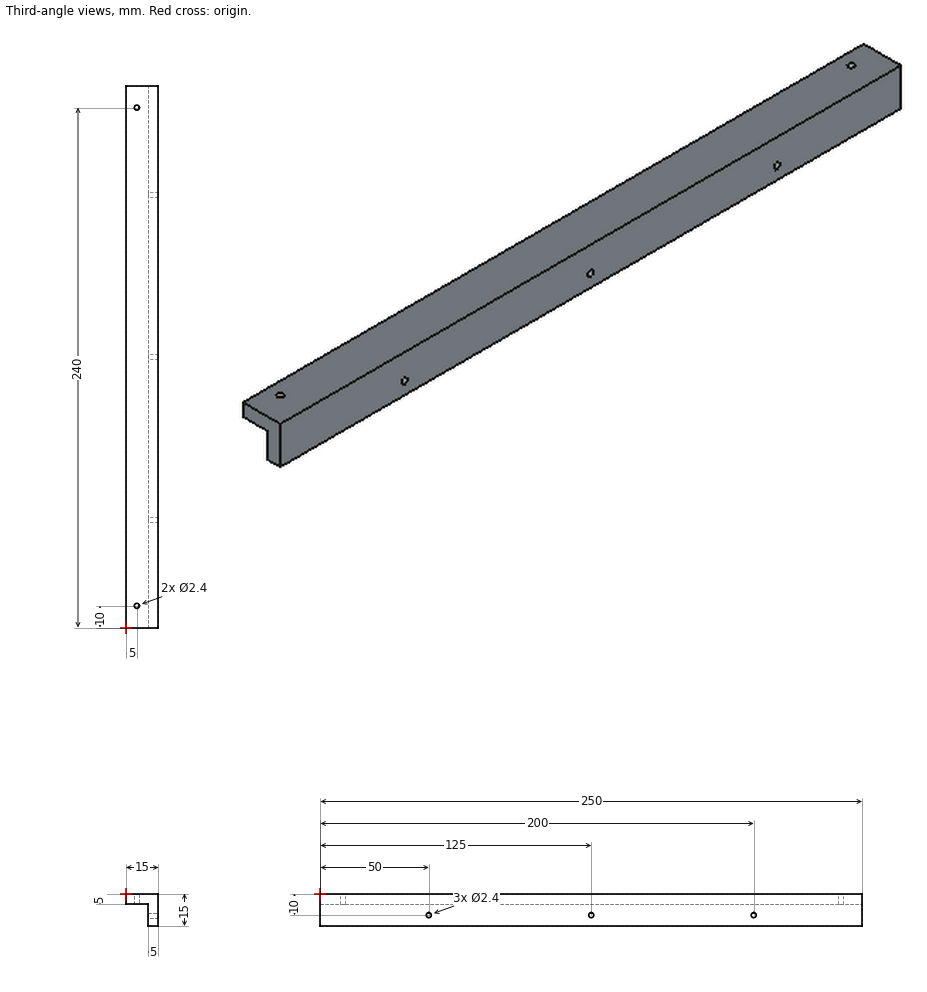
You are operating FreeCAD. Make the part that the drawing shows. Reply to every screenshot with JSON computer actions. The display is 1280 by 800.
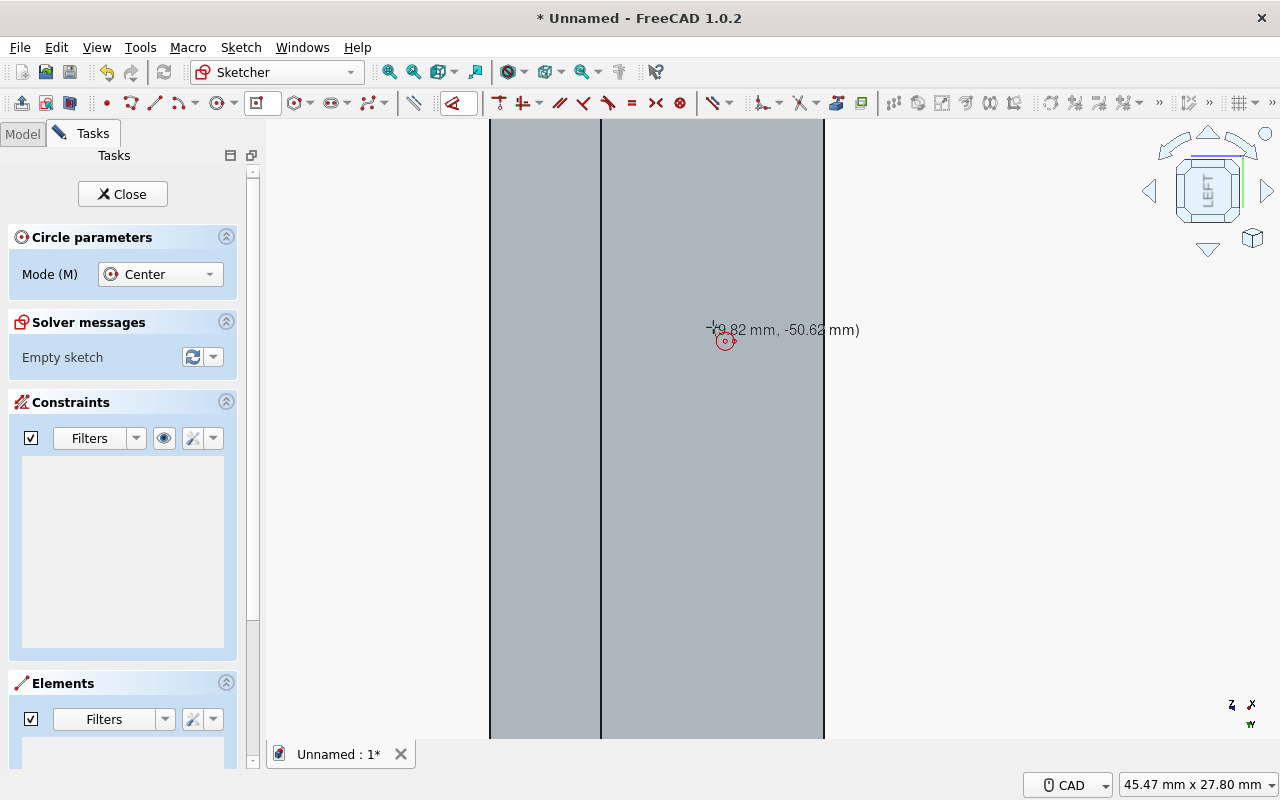
{"action": "scroll", "coordinate": [713, 327], "scroll_direction": "down", "scroll_amount": 12}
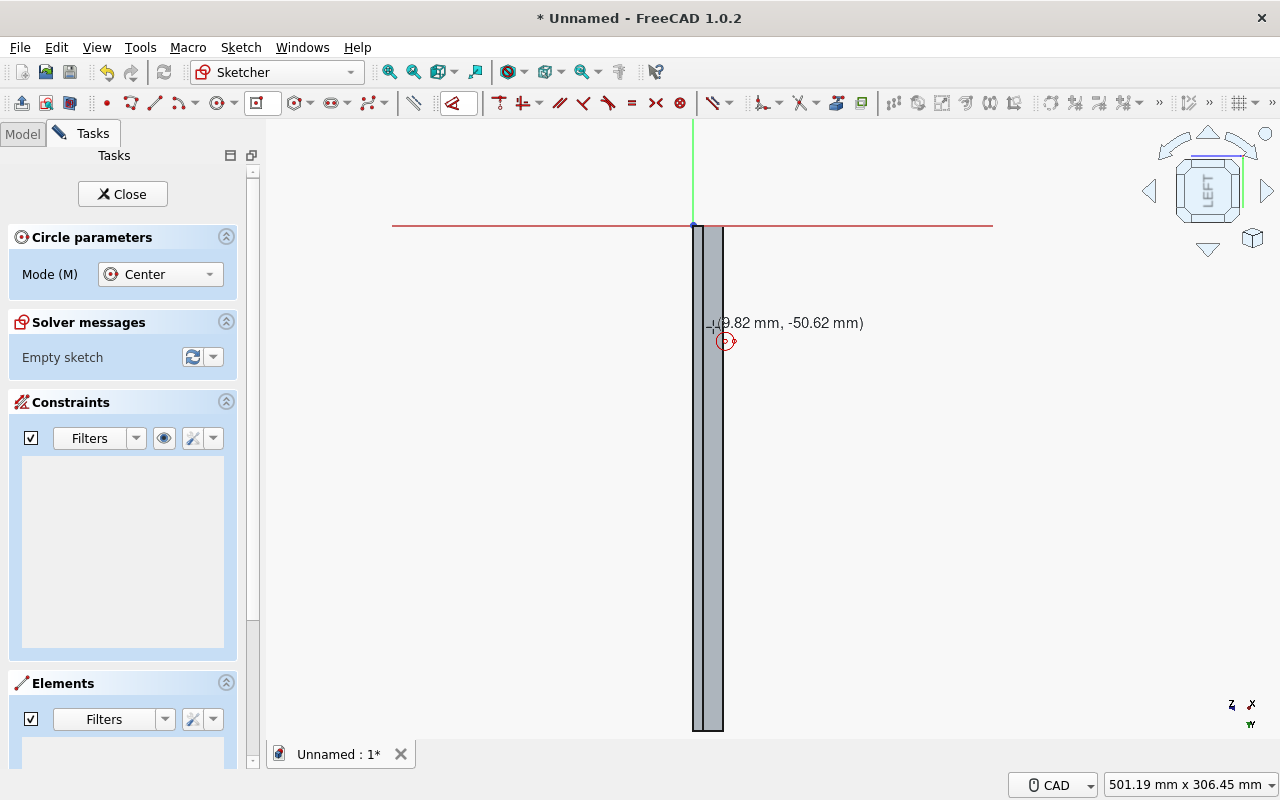
{"action": "left_click", "coordinate": [713, 327]}
{"action": "mouse_move", "coordinate": [715, 325]}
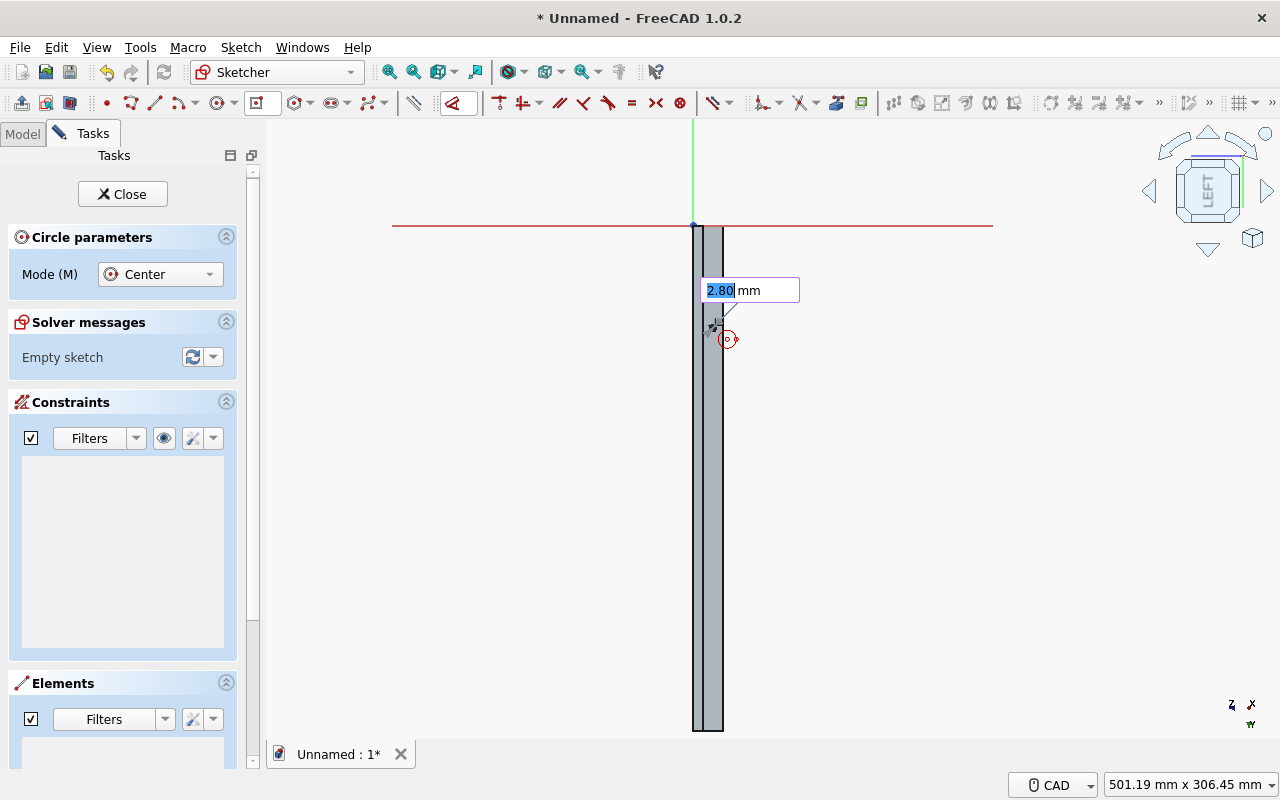
{"action": "type", "text": "2.4"}
{"action": "key", "text": "Return"}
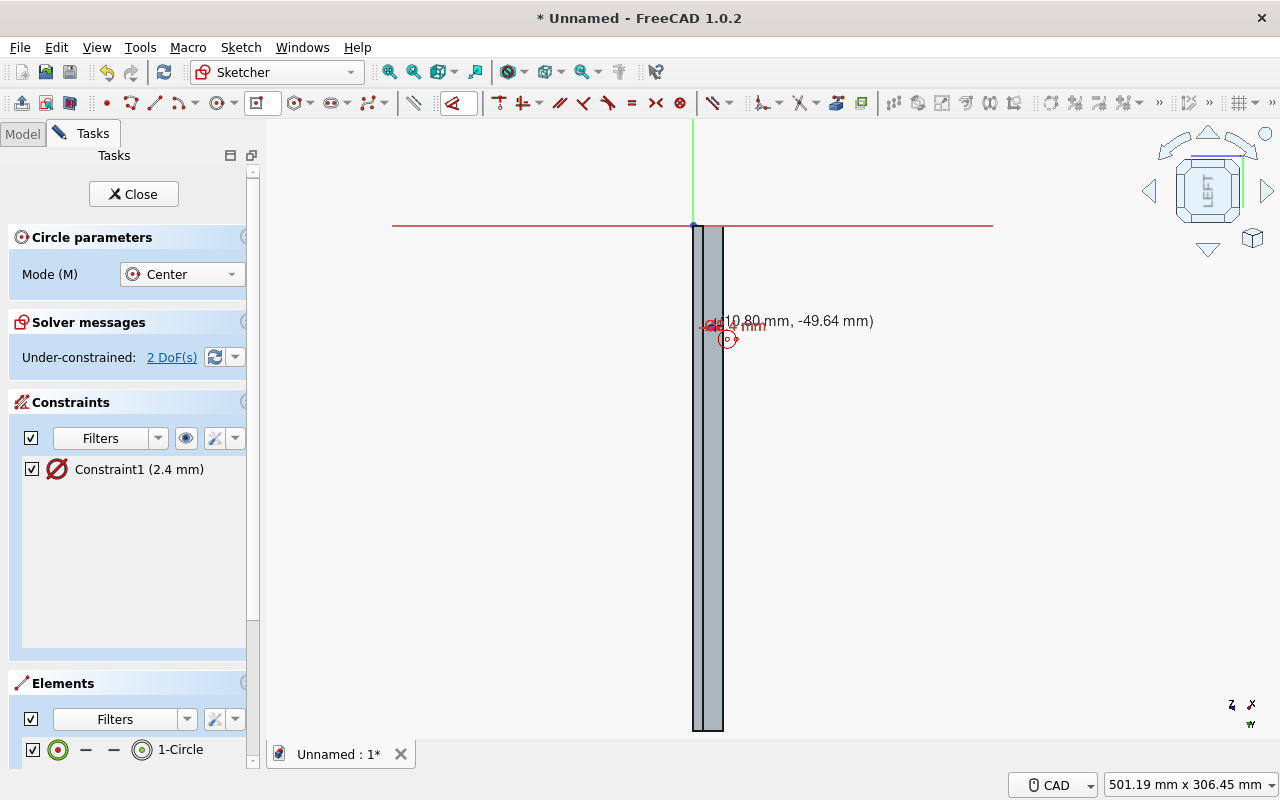
{"action": "scroll", "coordinate": [713, 478], "scroll_direction": "up", "scroll_amount": 12}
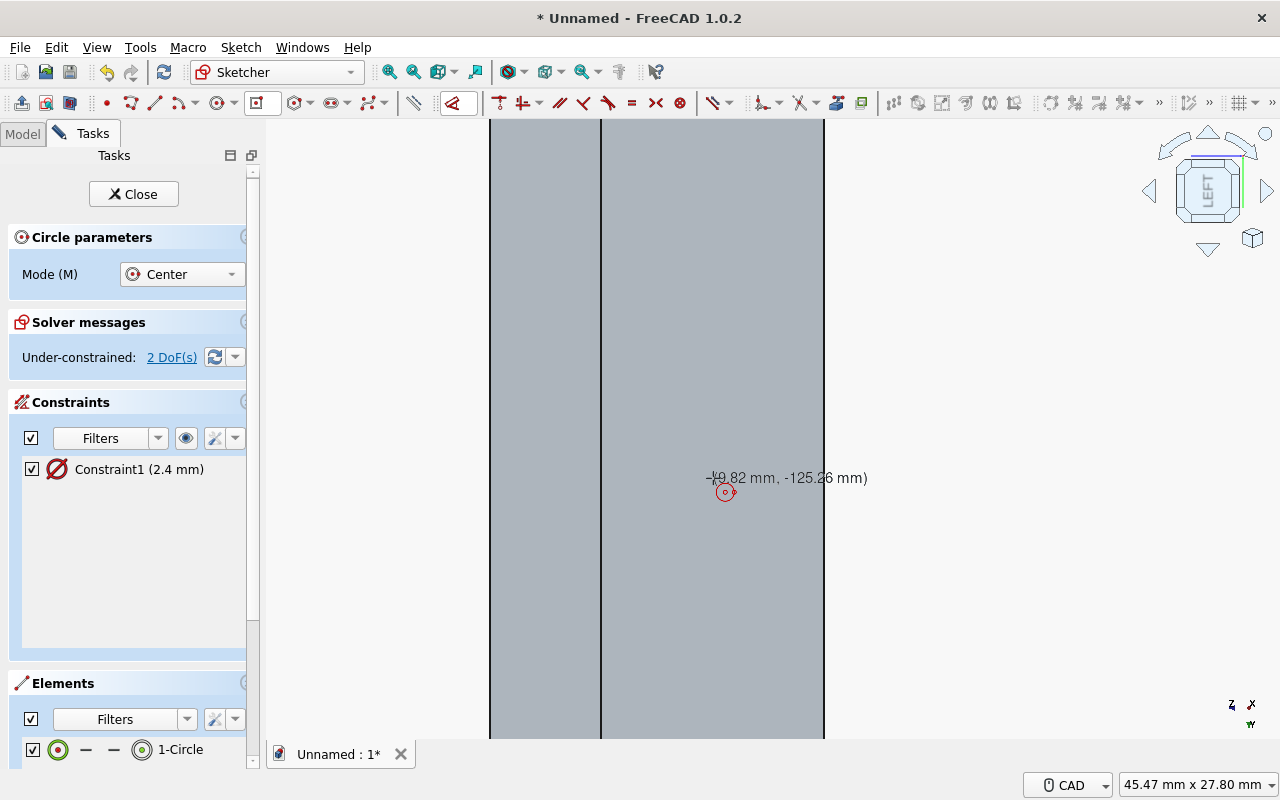
{"action": "scroll", "coordinate": [713, 478], "scroll_direction": "down", "scroll_amount": 12}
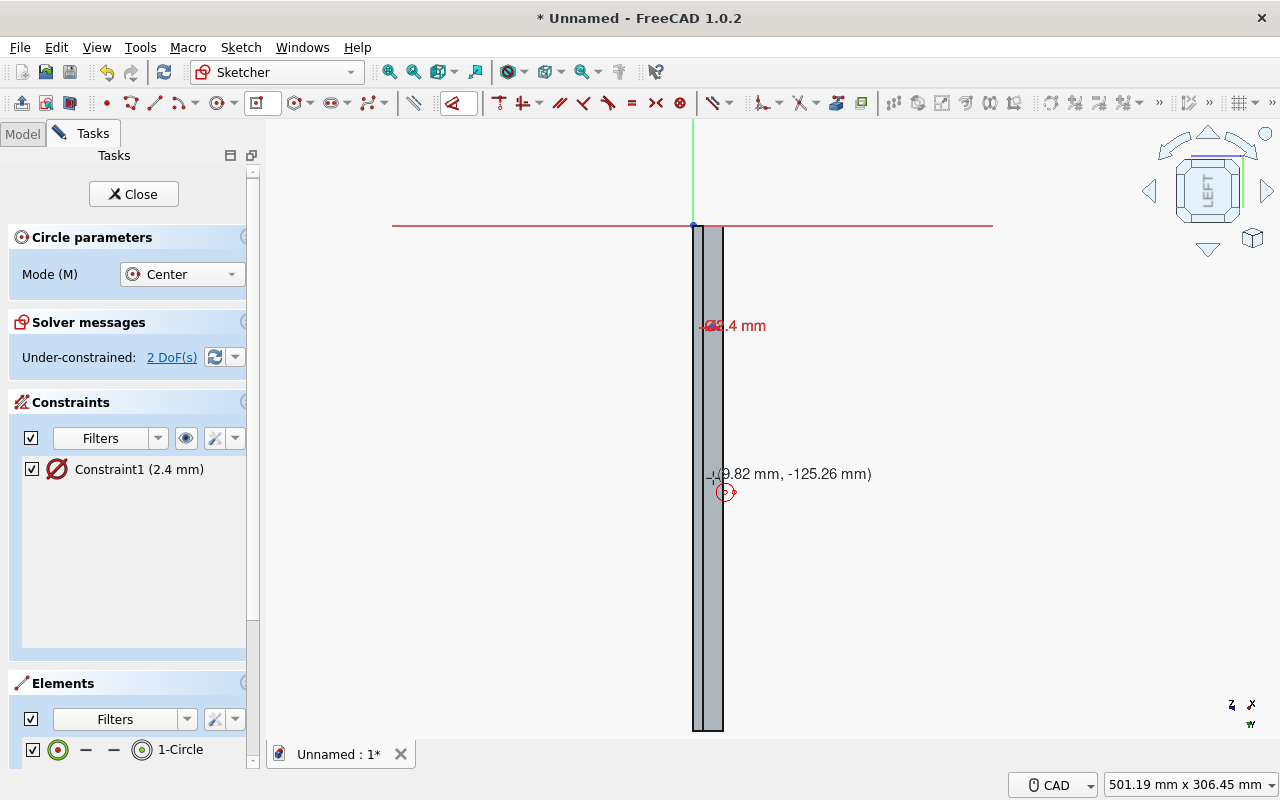
{"action": "left_click", "coordinate": [713, 478]}
{"action": "mouse_move", "coordinate": [715, 477]}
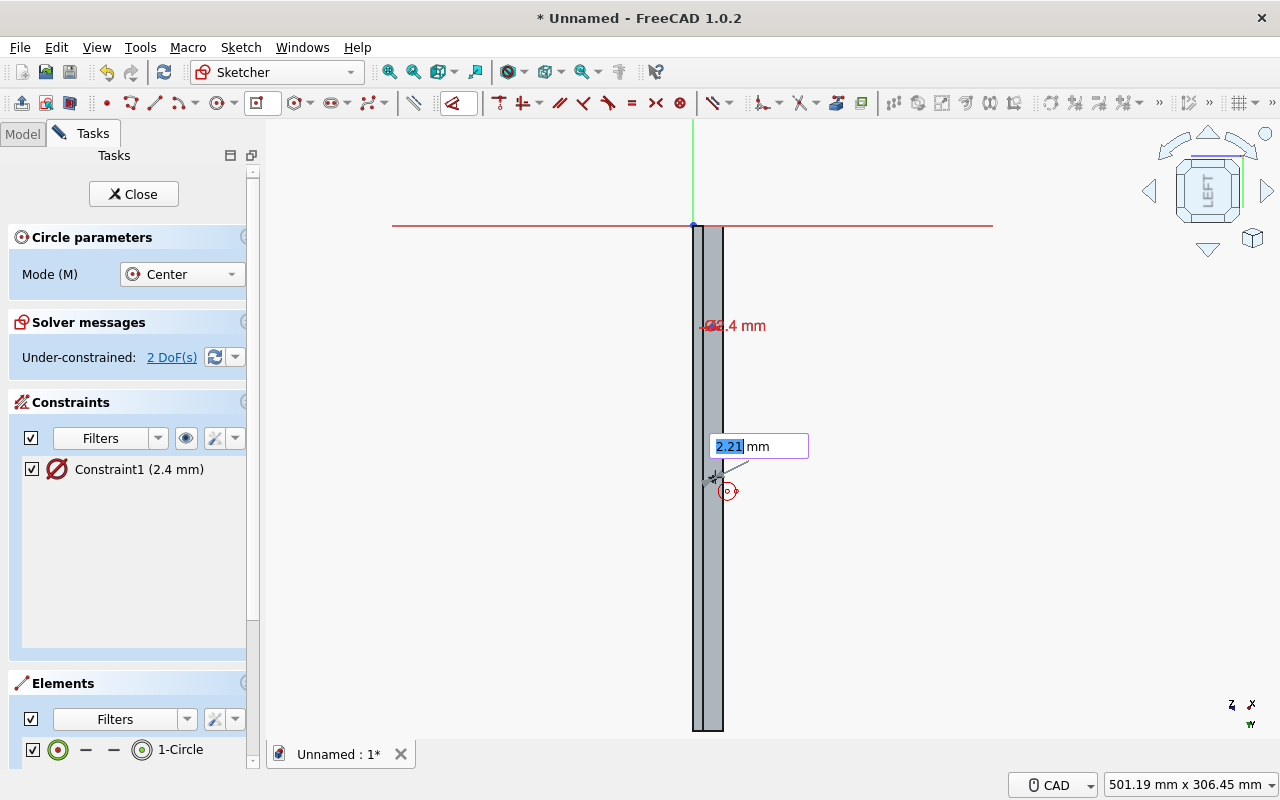
{"action": "type", "text": "2.4"}
{"action": "key", "text": "Return"}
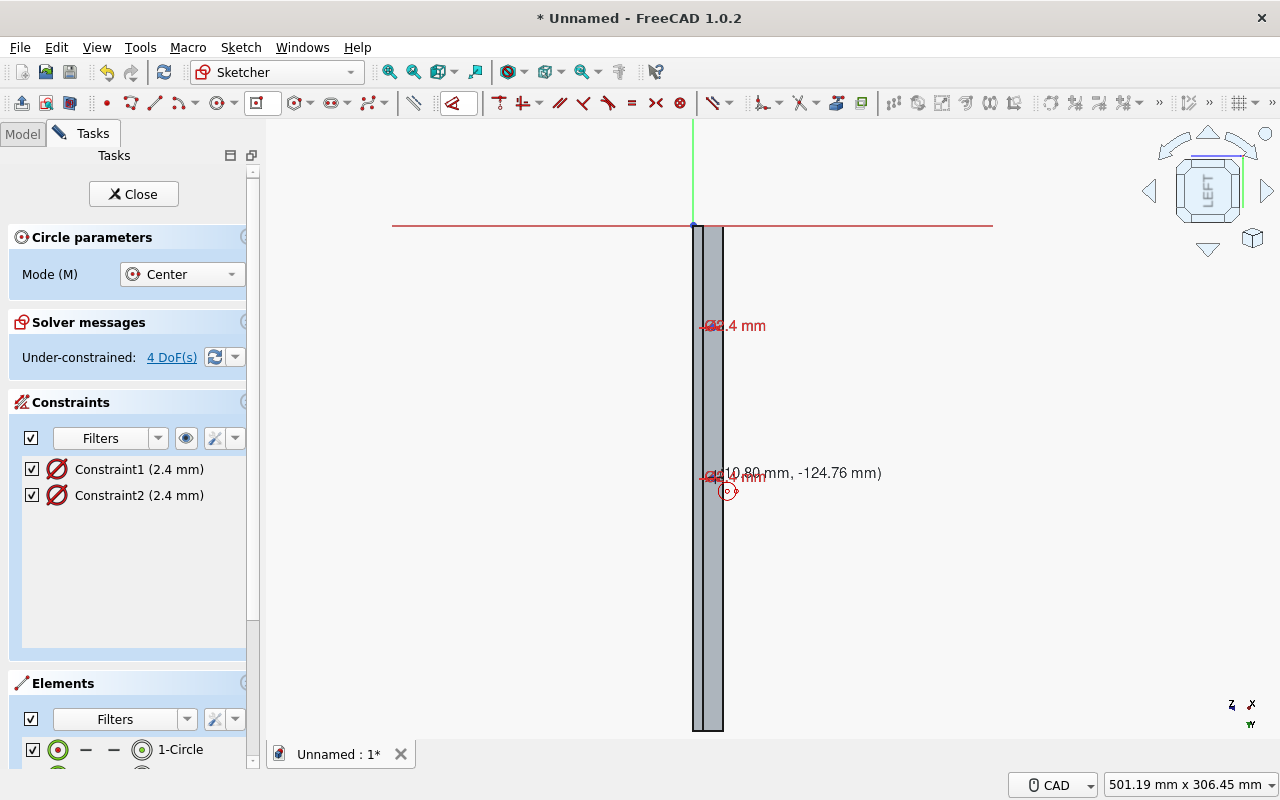
{"action": "scroll", "coordinate": [713, 630], "scroll_direction": "up", "scroll_amount": 12}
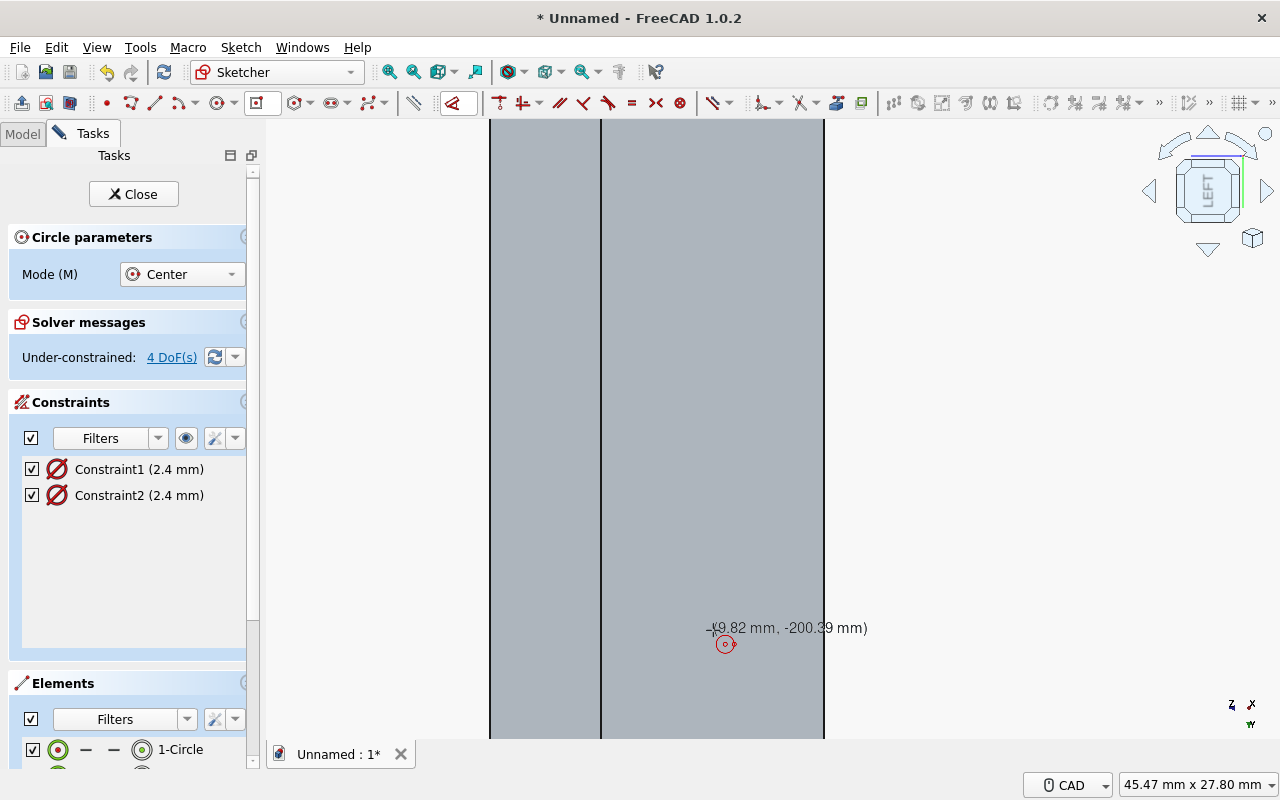
{"action": "scroll", "coordinate": [713, 631], "scroll_direction": "down", "scroll_amount": 12}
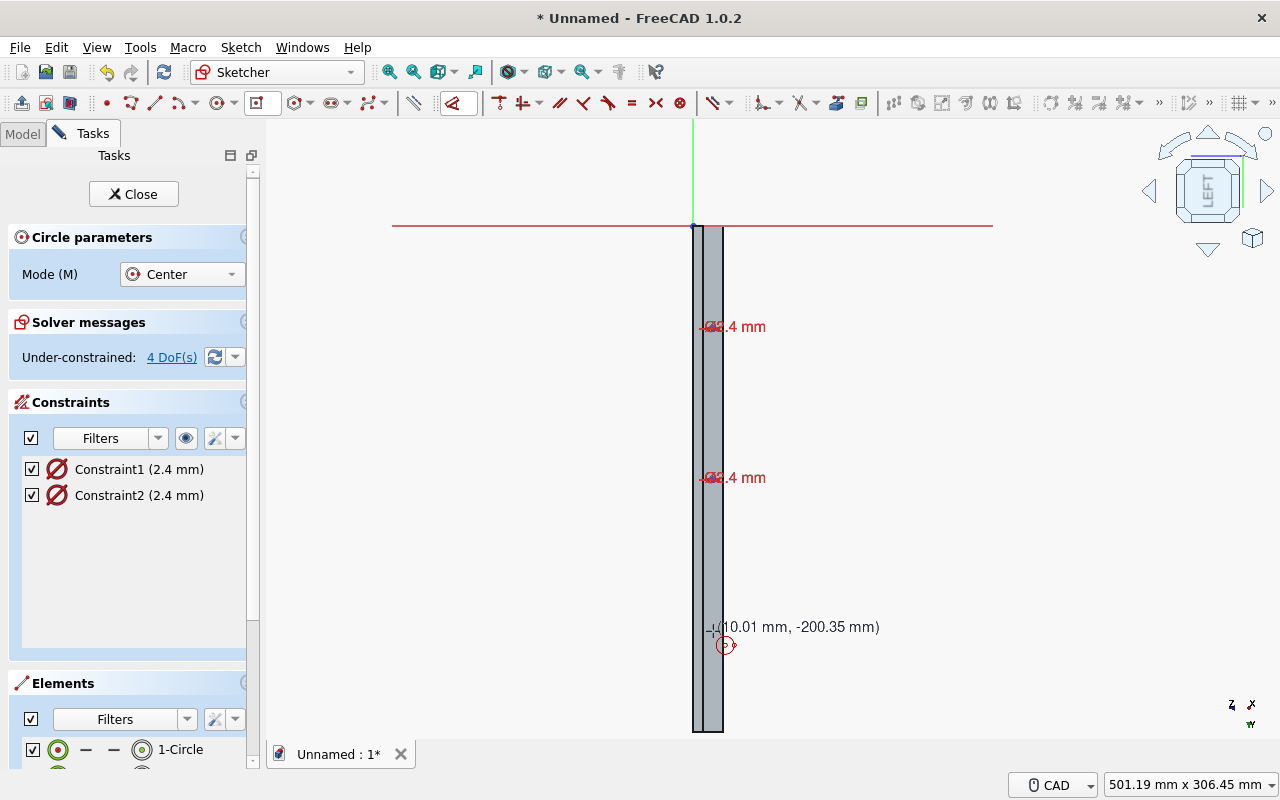
{"action": "left_click", "coordinate": [713, 631]}
{"action": "mouse_move", "coordinate": [715, 629]}